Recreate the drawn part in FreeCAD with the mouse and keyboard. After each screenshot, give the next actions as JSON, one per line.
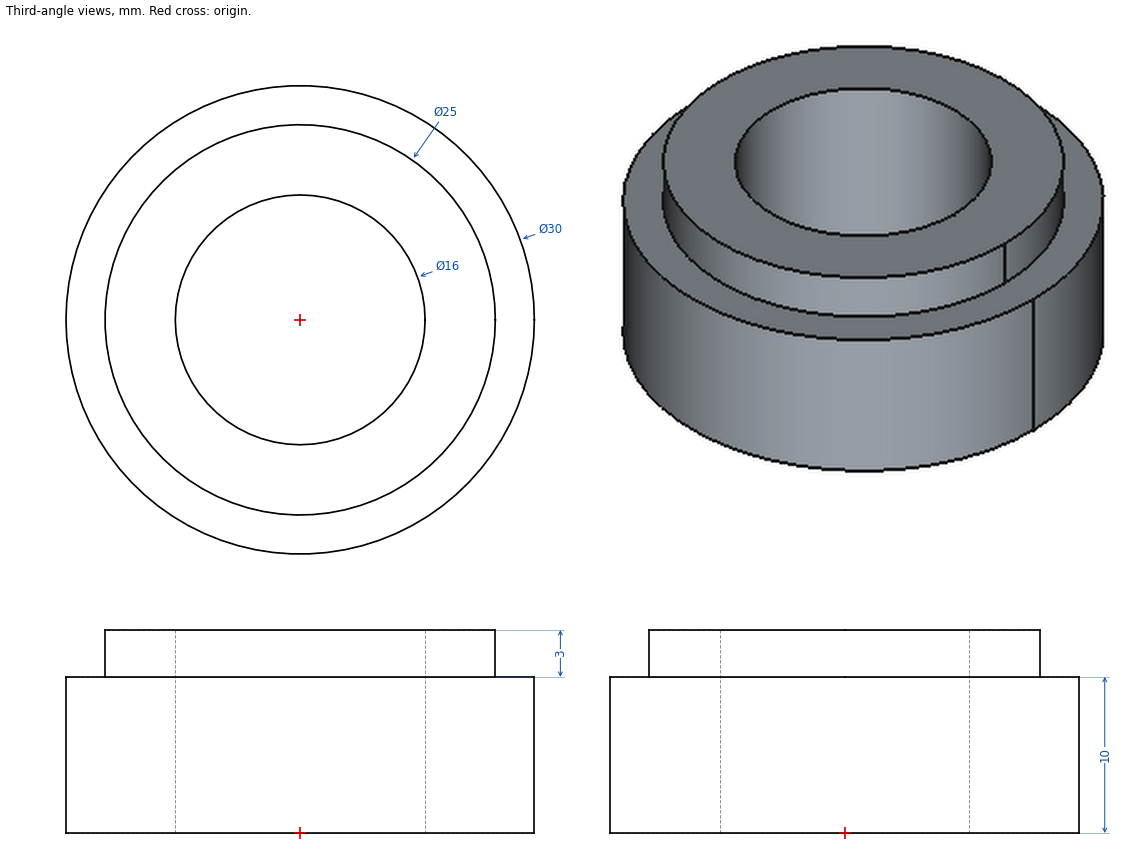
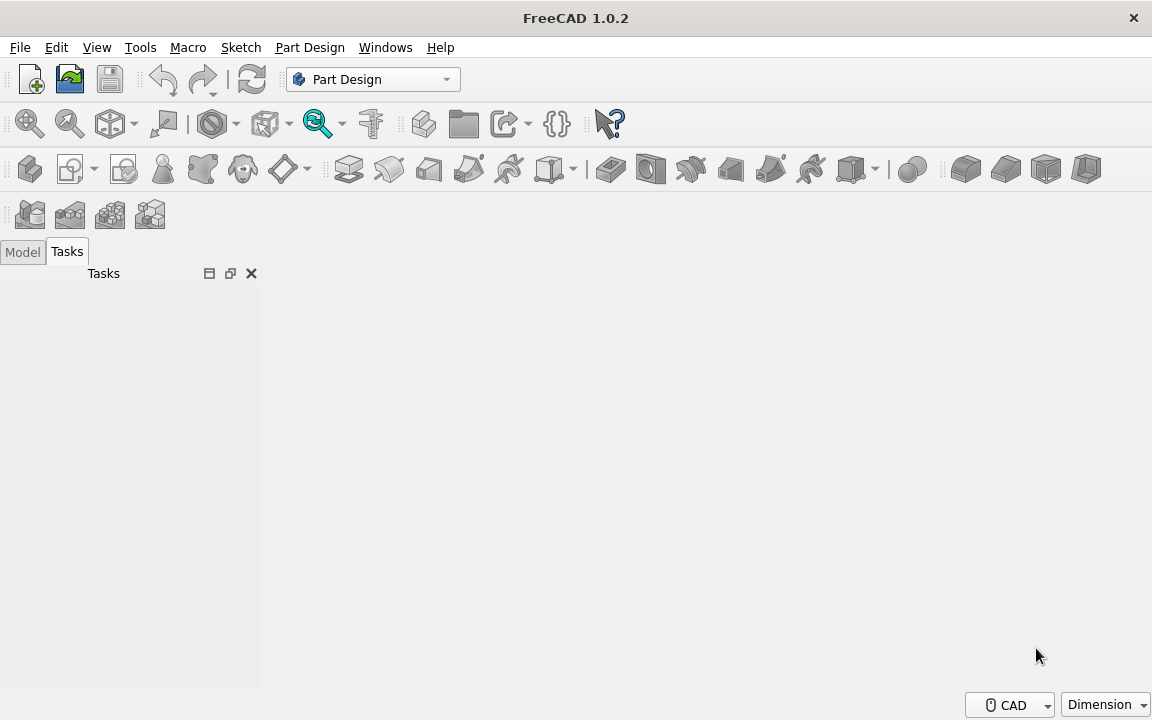
{"action": "key", "text": "ctrl+n"}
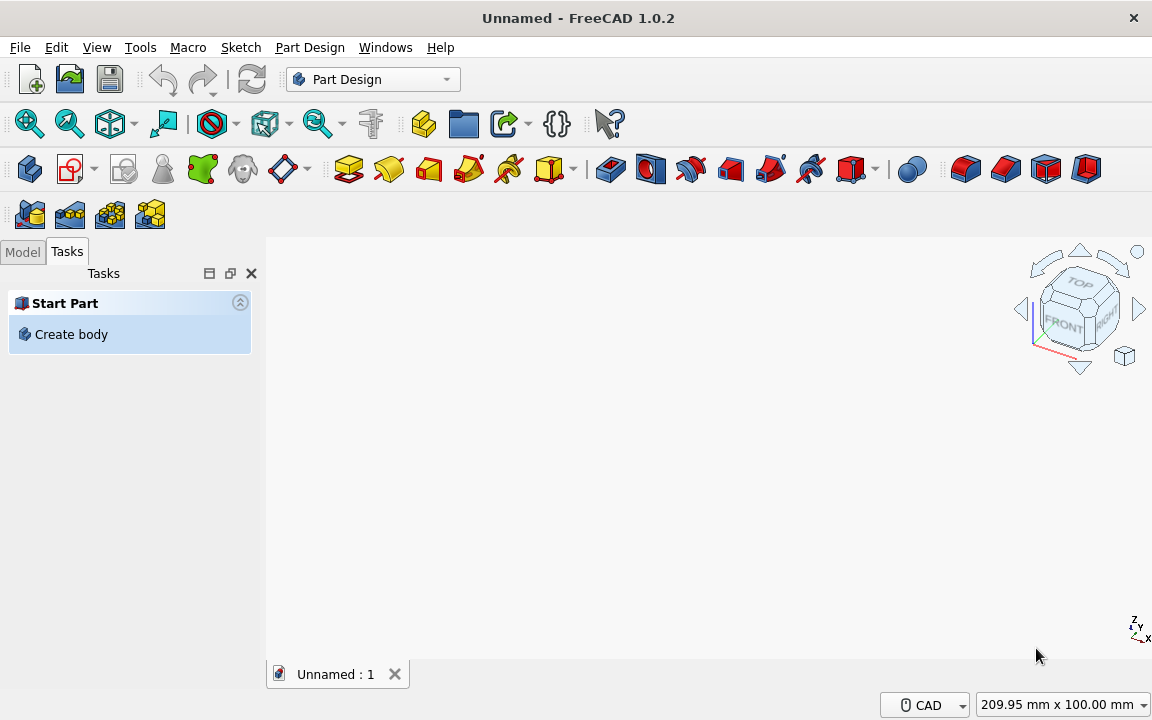
{"action": "left_click", "coordinate": [70, 170]}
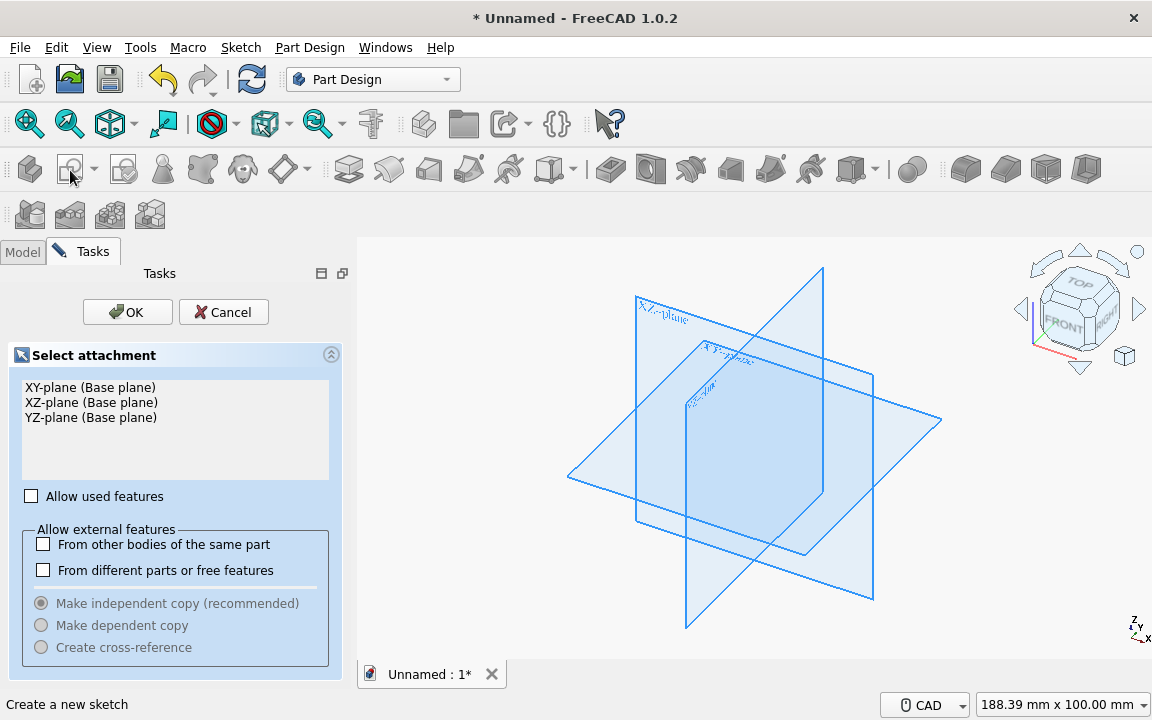
{"action": "left_click", "coordinate": [82, 388]}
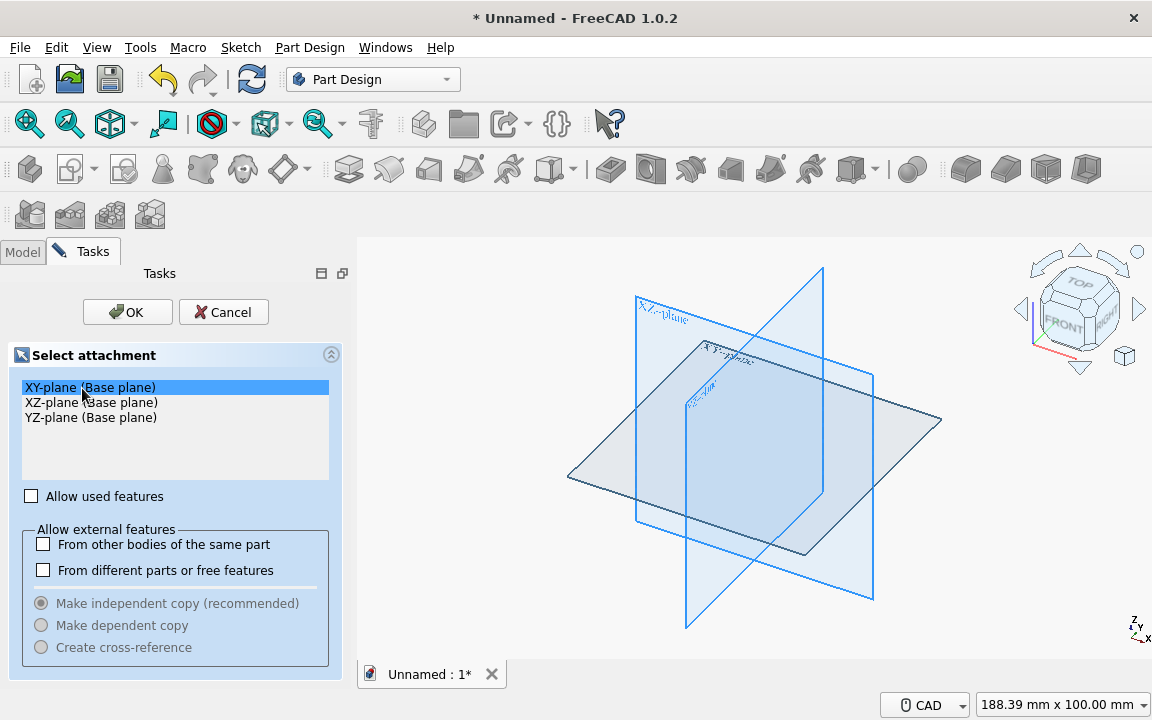
{"action": "left_click", "coordinate": [128, 312]}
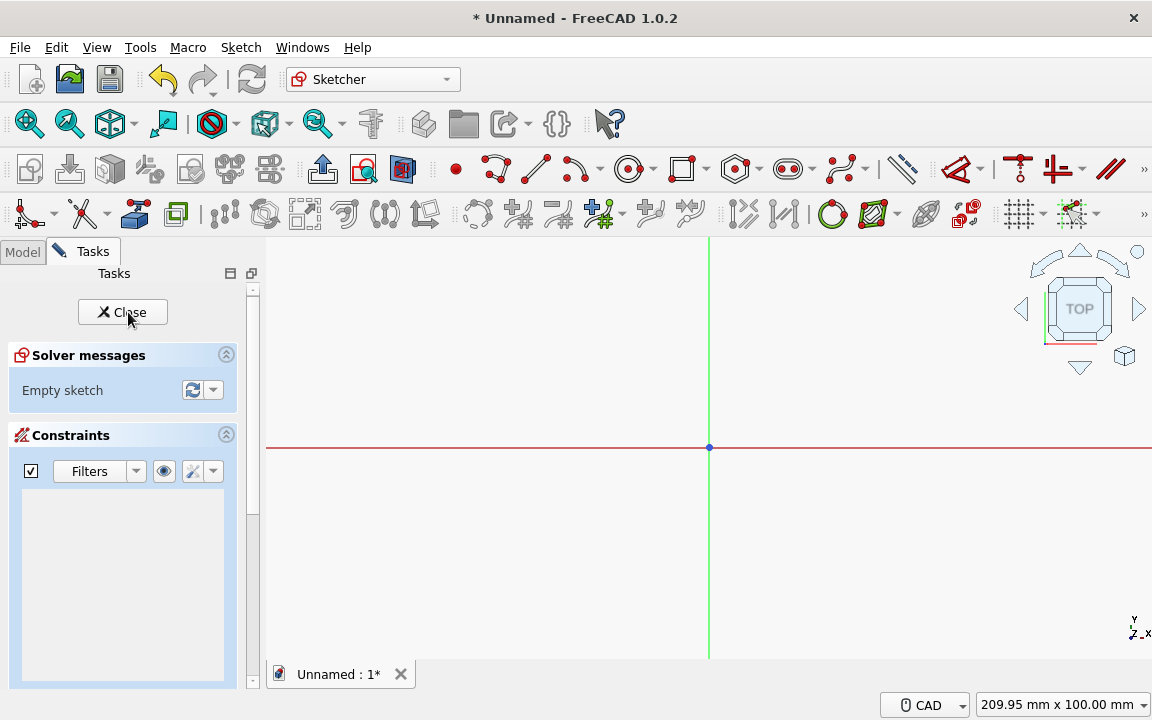
{"action": "scroll", "coordinate": [765, 448], "scroll_direction": "up", "scroll_amount": 4}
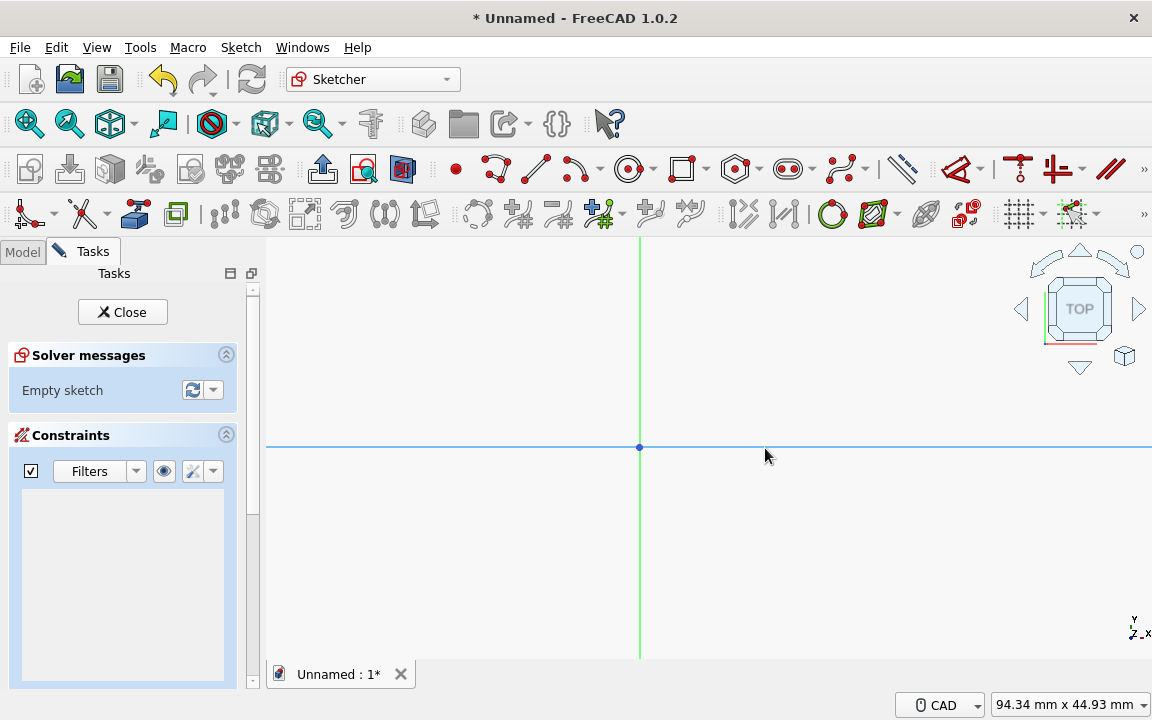
{"action": "left_click", "coordinate": [630, 170]}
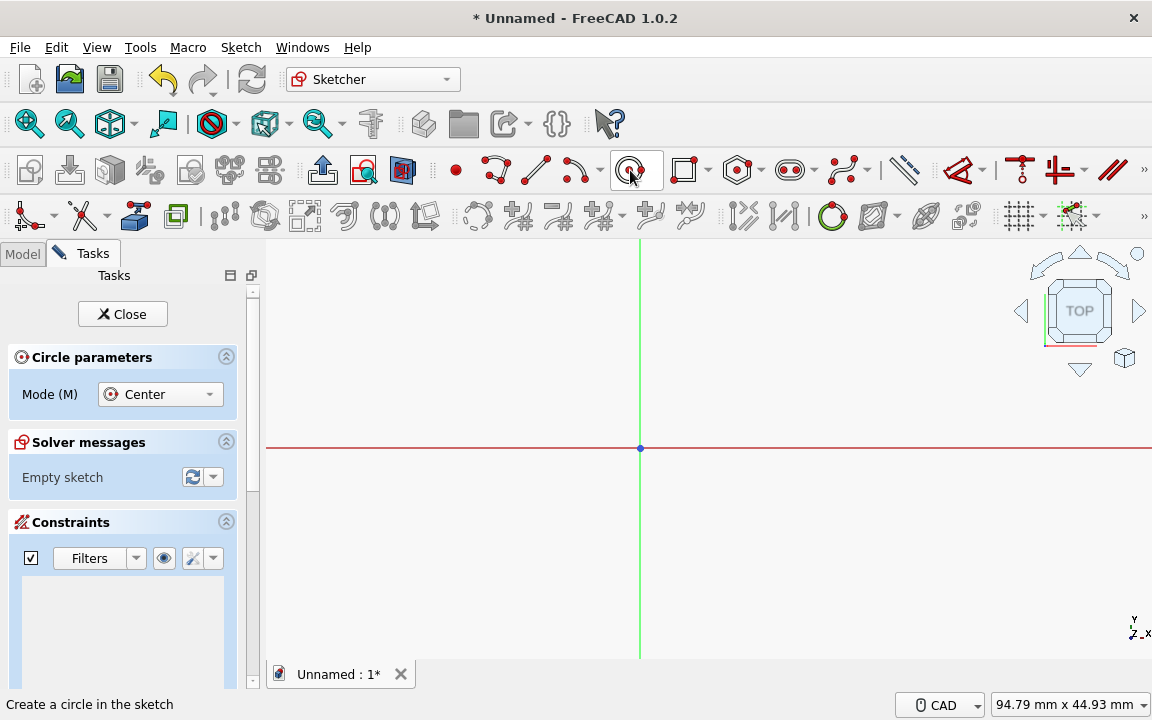
{"action": "left_click", "coordinate": [640, 448]}
{"action": "left_click", "coordinate": [739, 349]}
{"action": "key", "text": "Escape"}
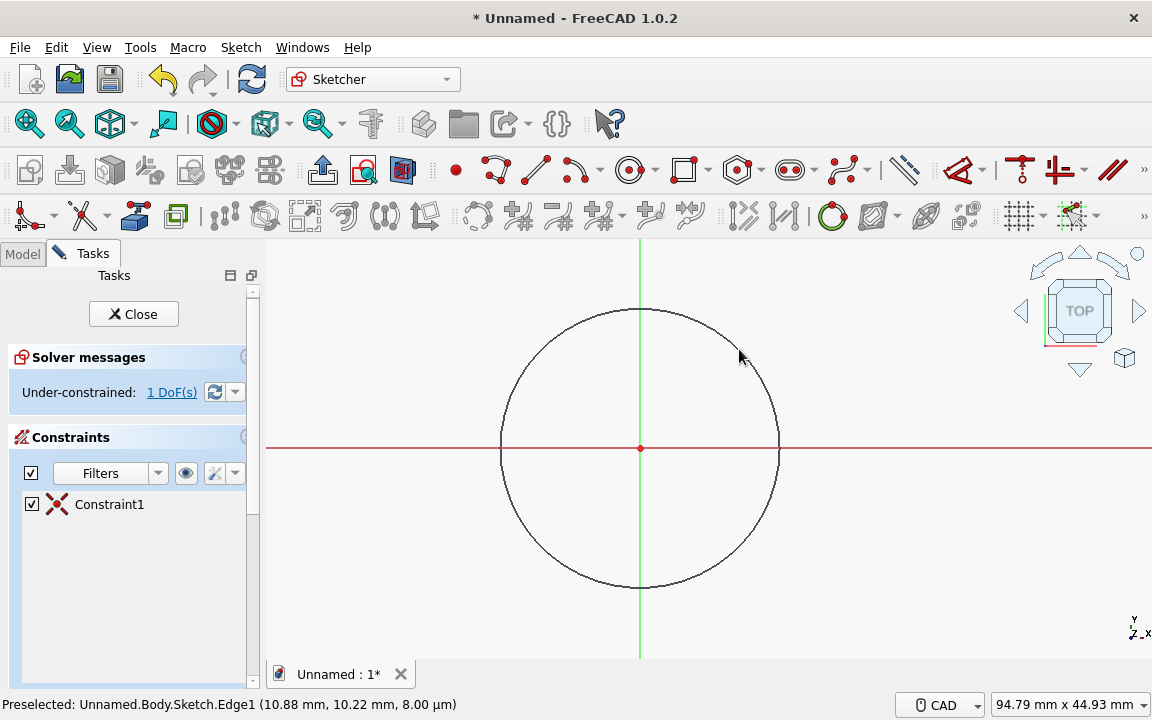
{"action": "left_click", "coordinate": [738, 349]}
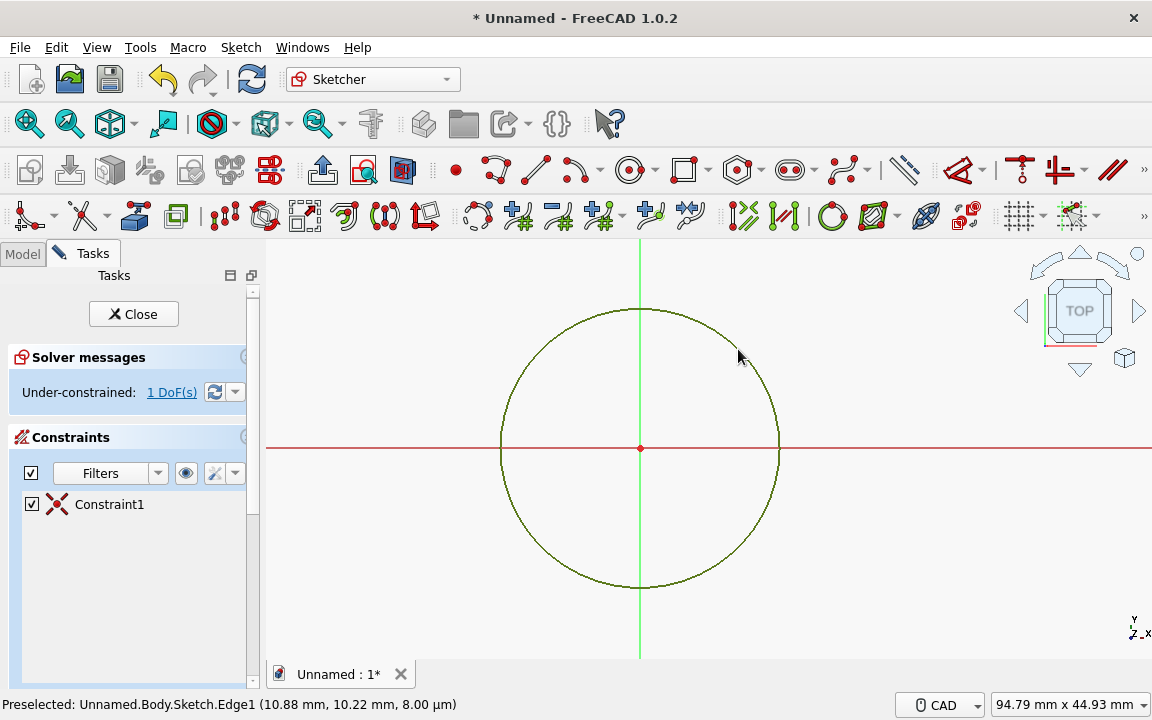
{"action": "key", "text": "k o"}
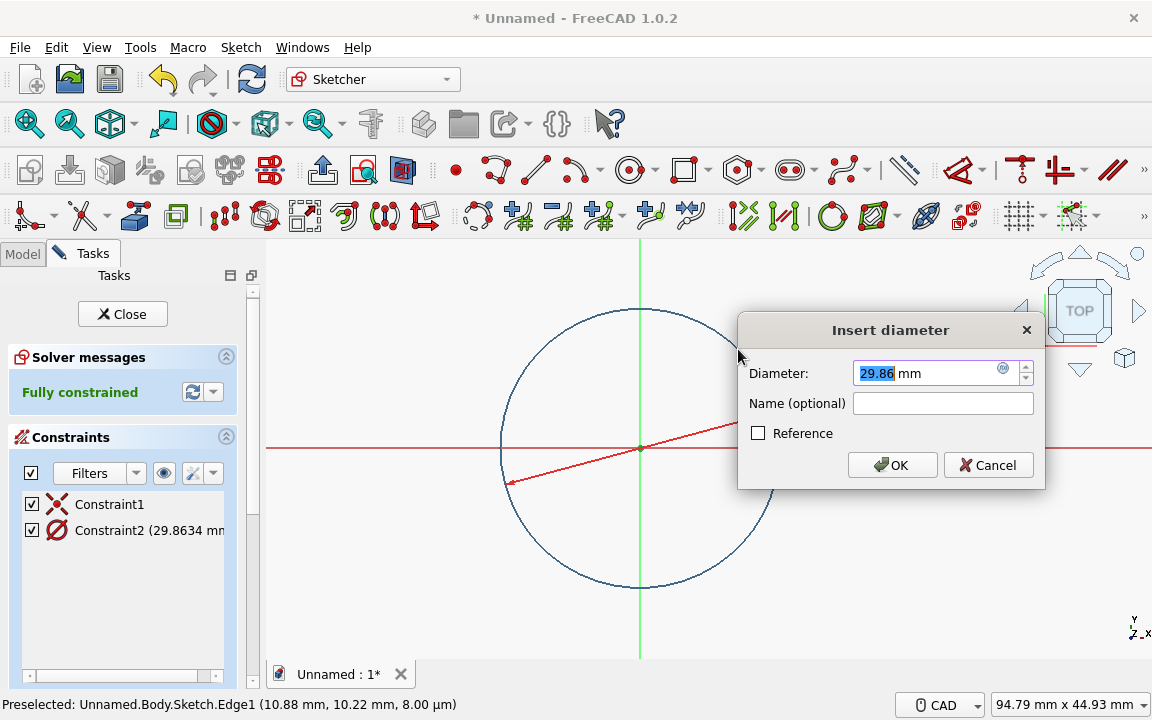
{"action": "type", "text": "30"}
{"action": "key", "text": "Return"}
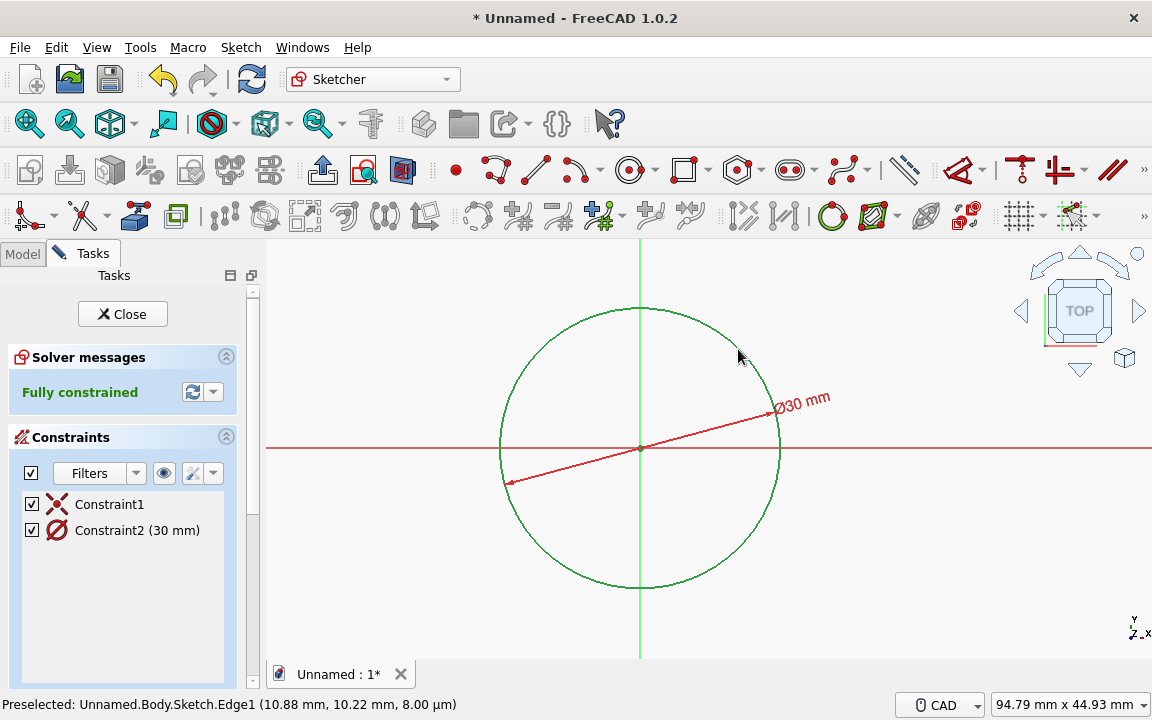
{"action": "left_click", "coordinate": [123, 314]}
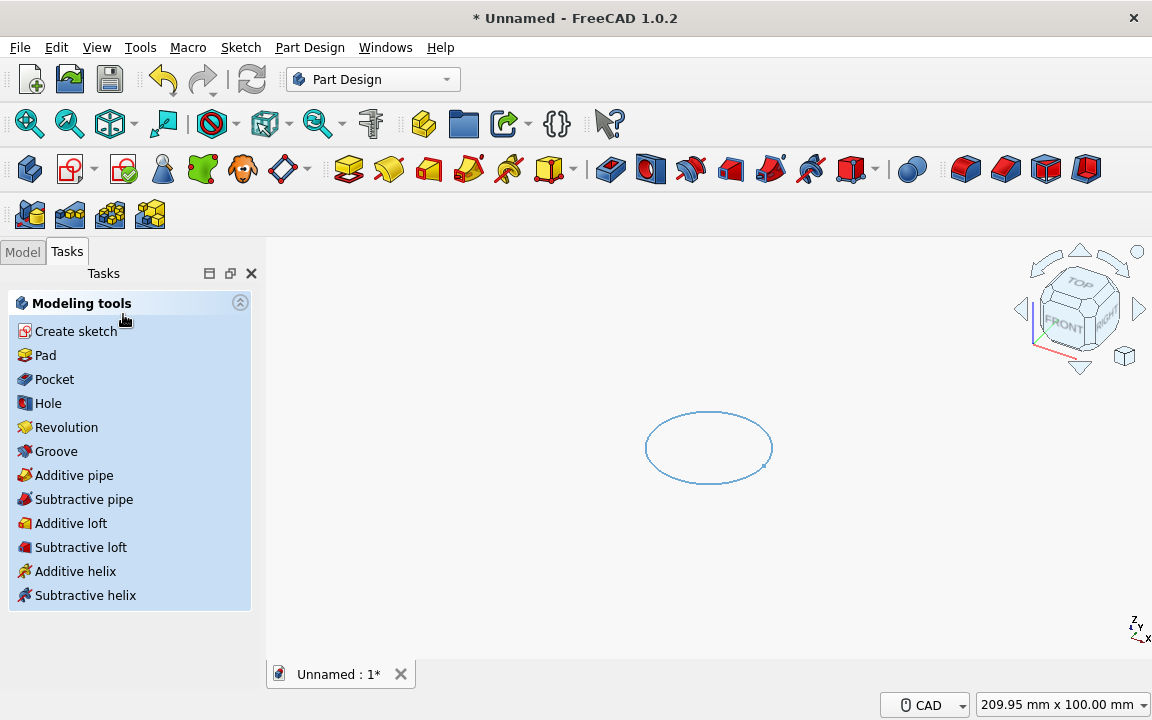
{"action": "left_click", "coordinate": [350, 170]}